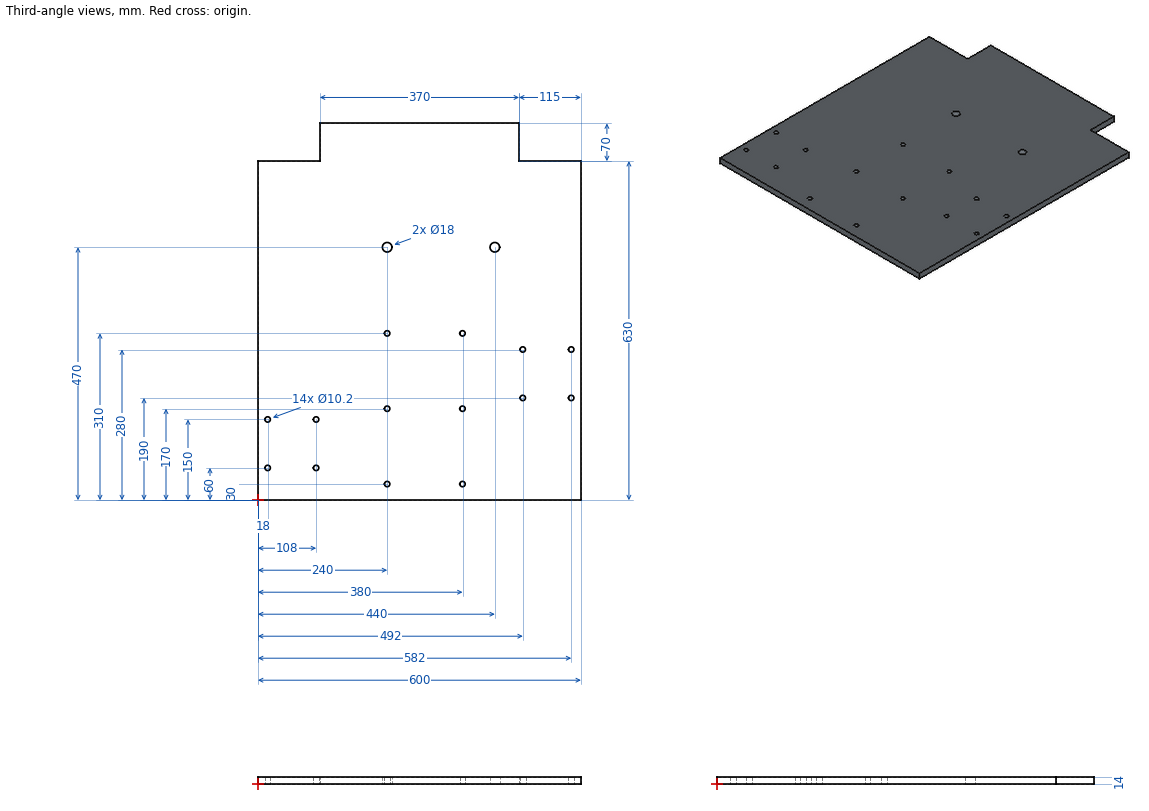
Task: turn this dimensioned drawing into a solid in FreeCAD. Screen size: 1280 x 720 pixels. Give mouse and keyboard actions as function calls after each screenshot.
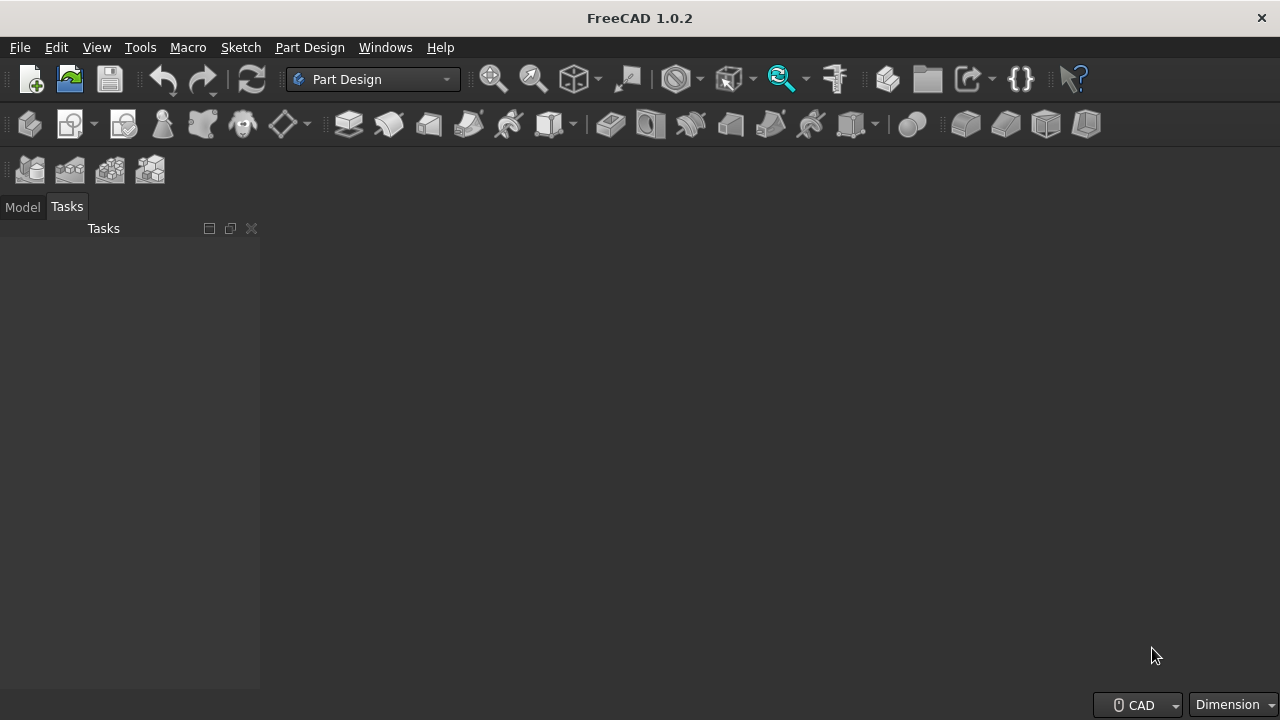
click(30, 80)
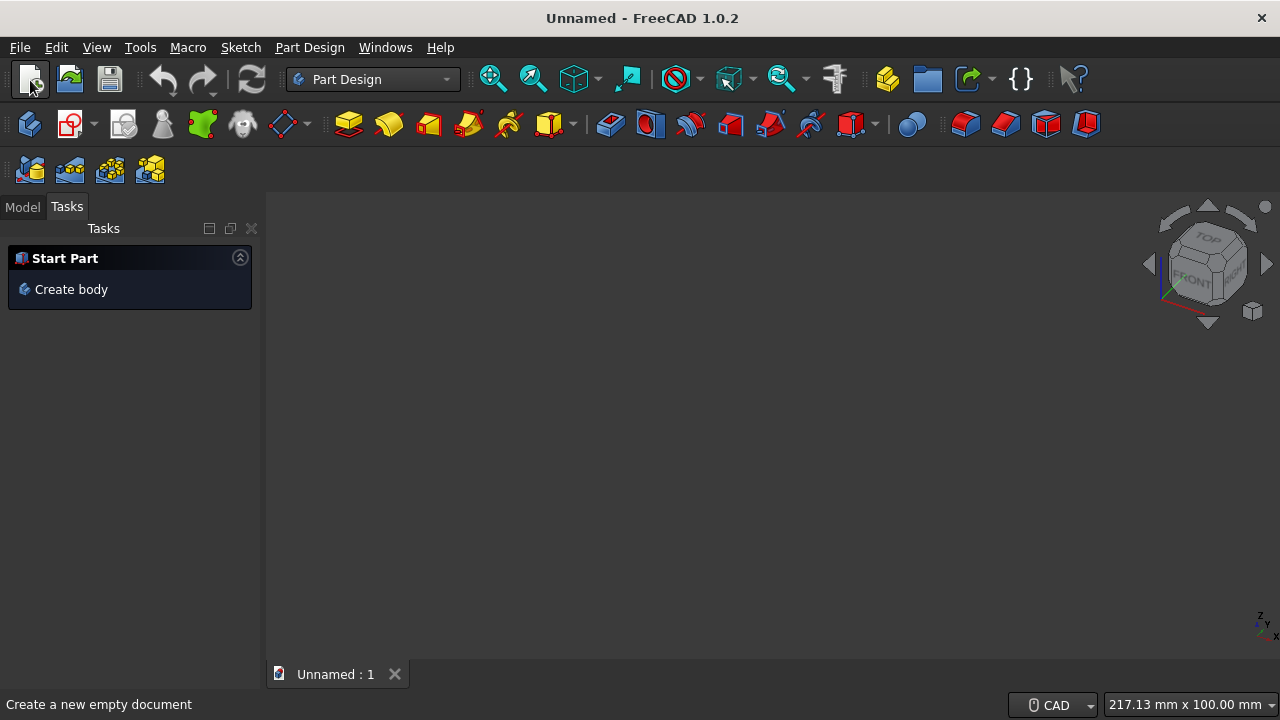
click(70, 124)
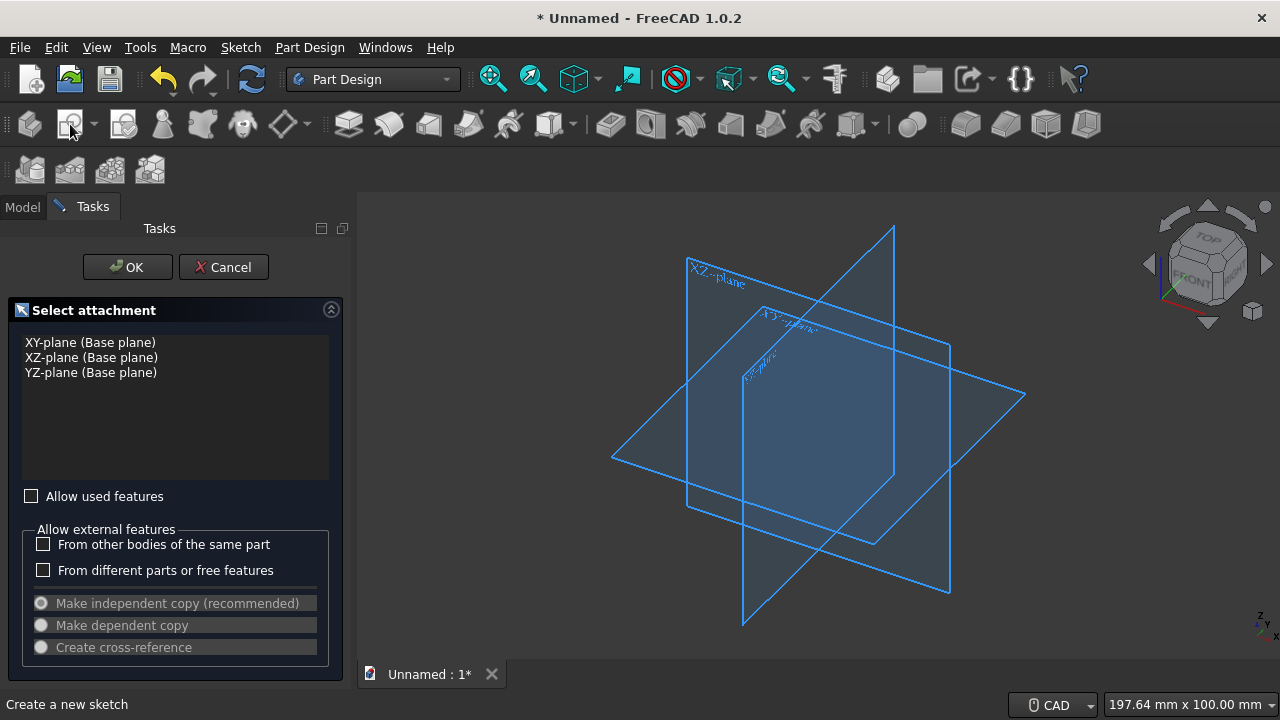
click(82, 342)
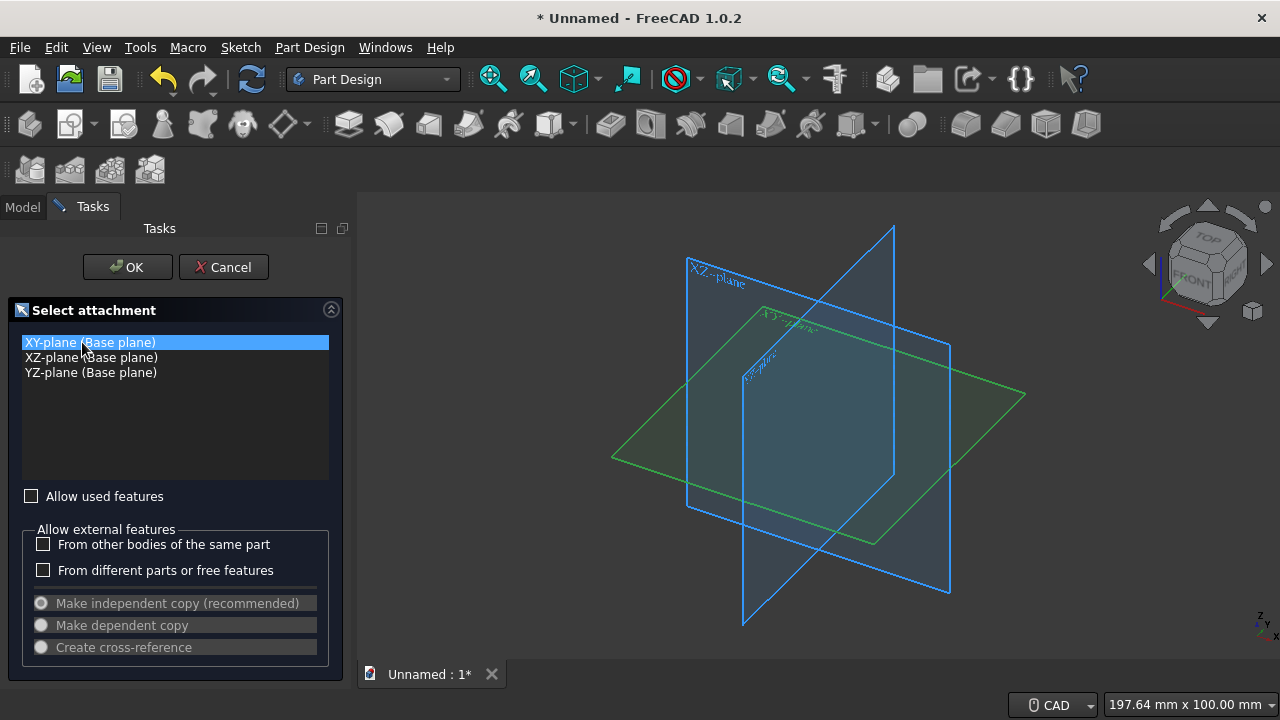
click(128, 267)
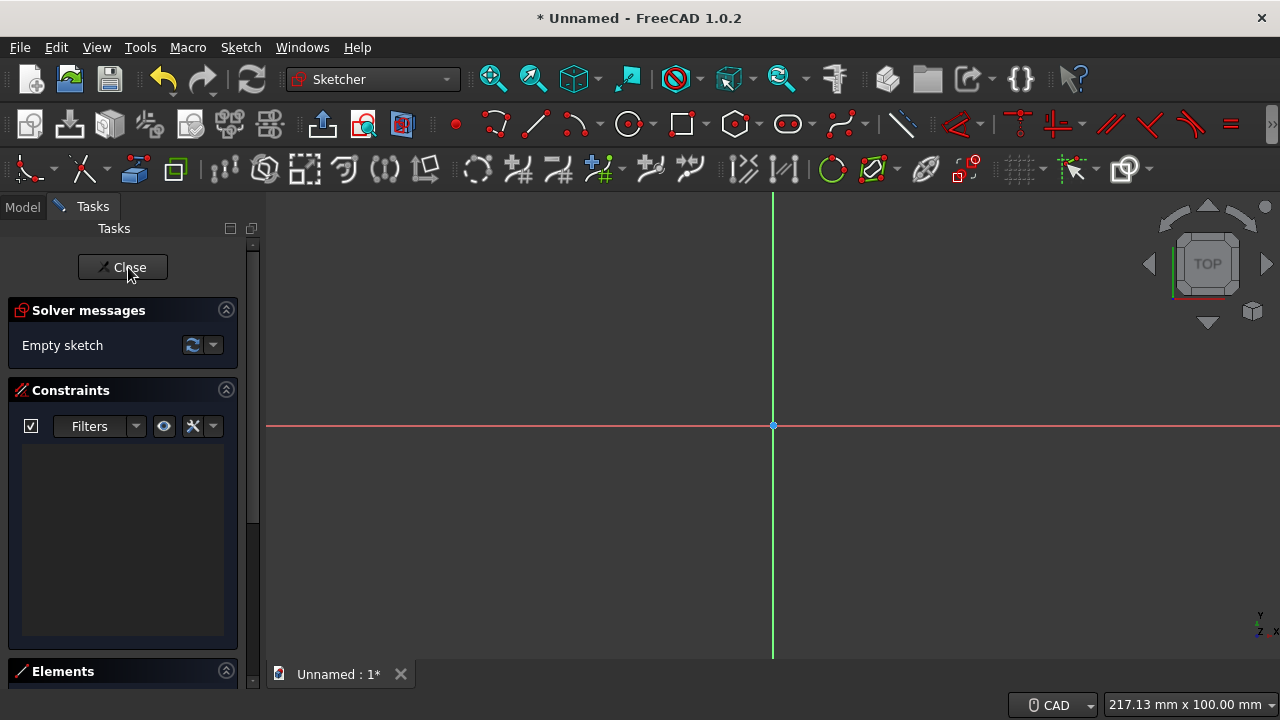
scroll(558, 589, down, 12)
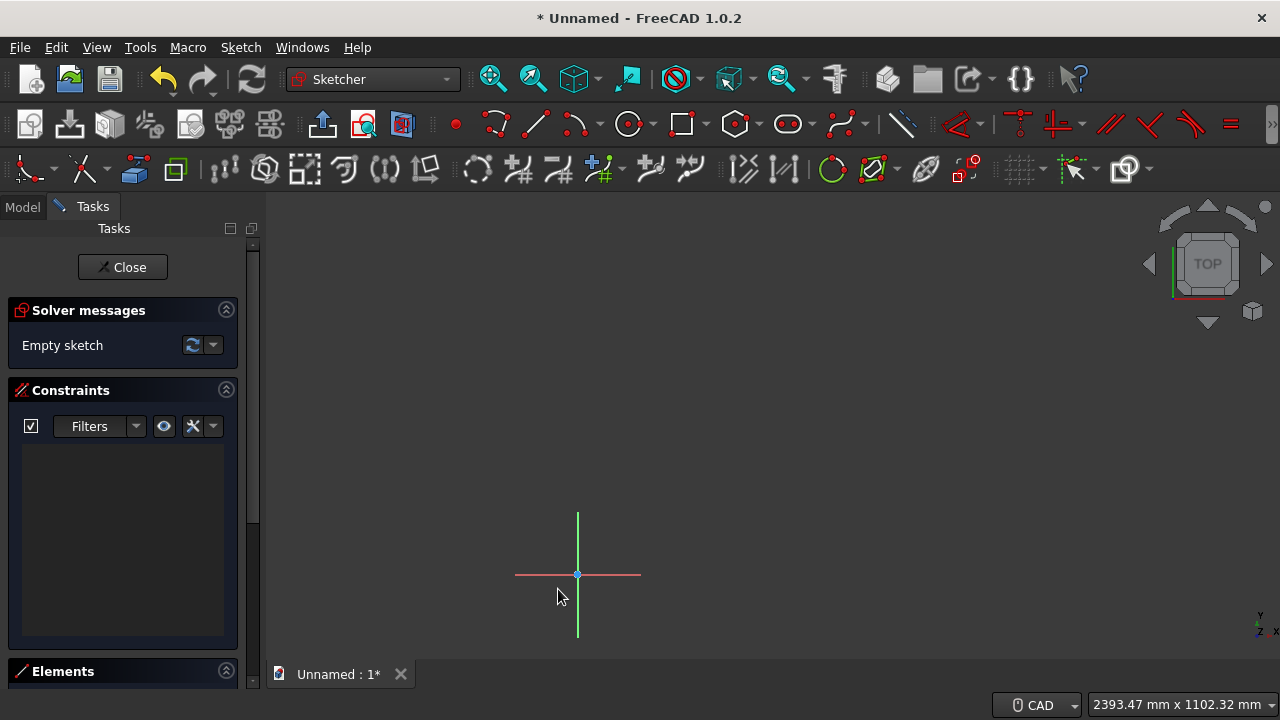
click(496, 124)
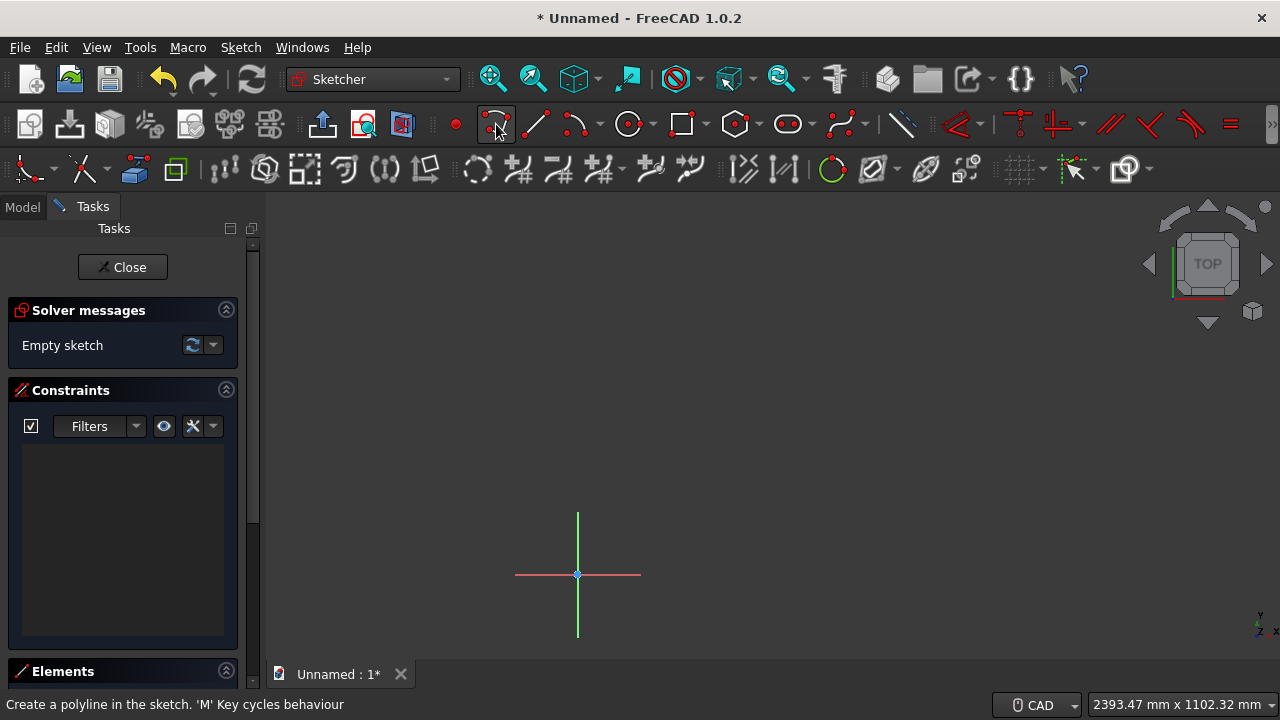
click(578, 575)
click(832, 566)
click(832, 308)
click(783, 308)
click(783, 278)
click(626, 278)
click(626, 308)
click(587, 308)
click(578, 575)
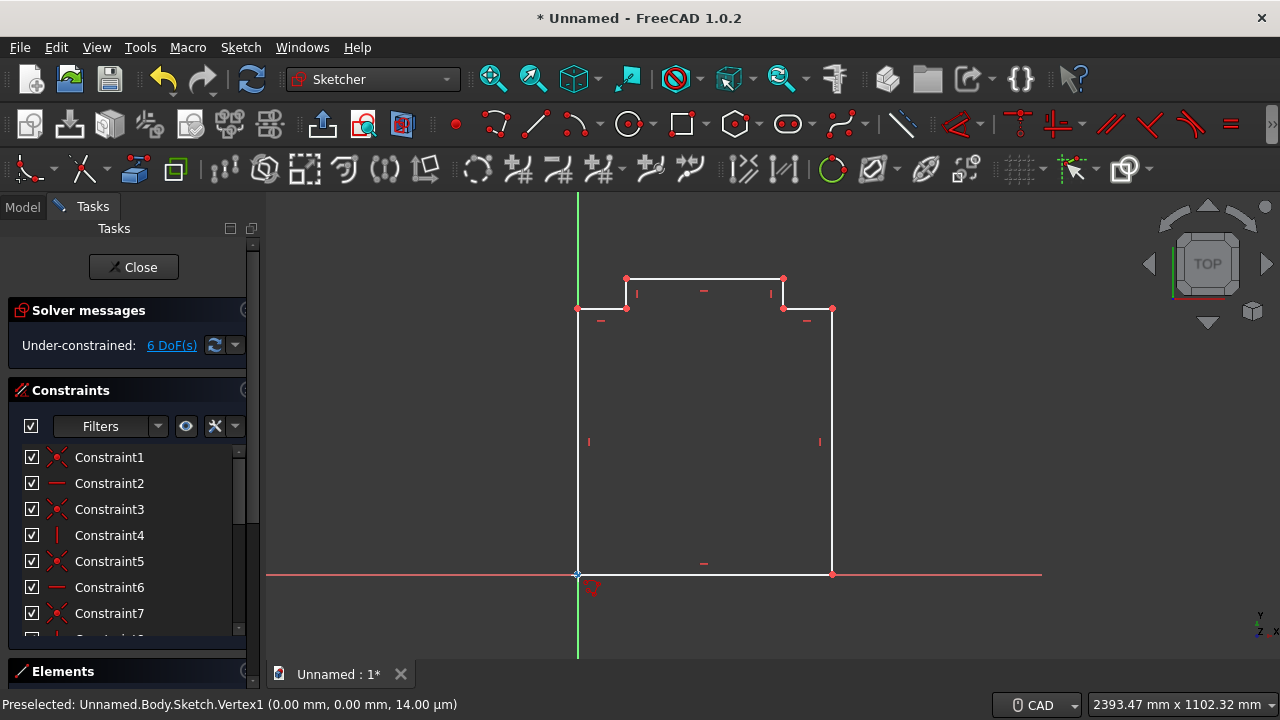
key(g)
key(c)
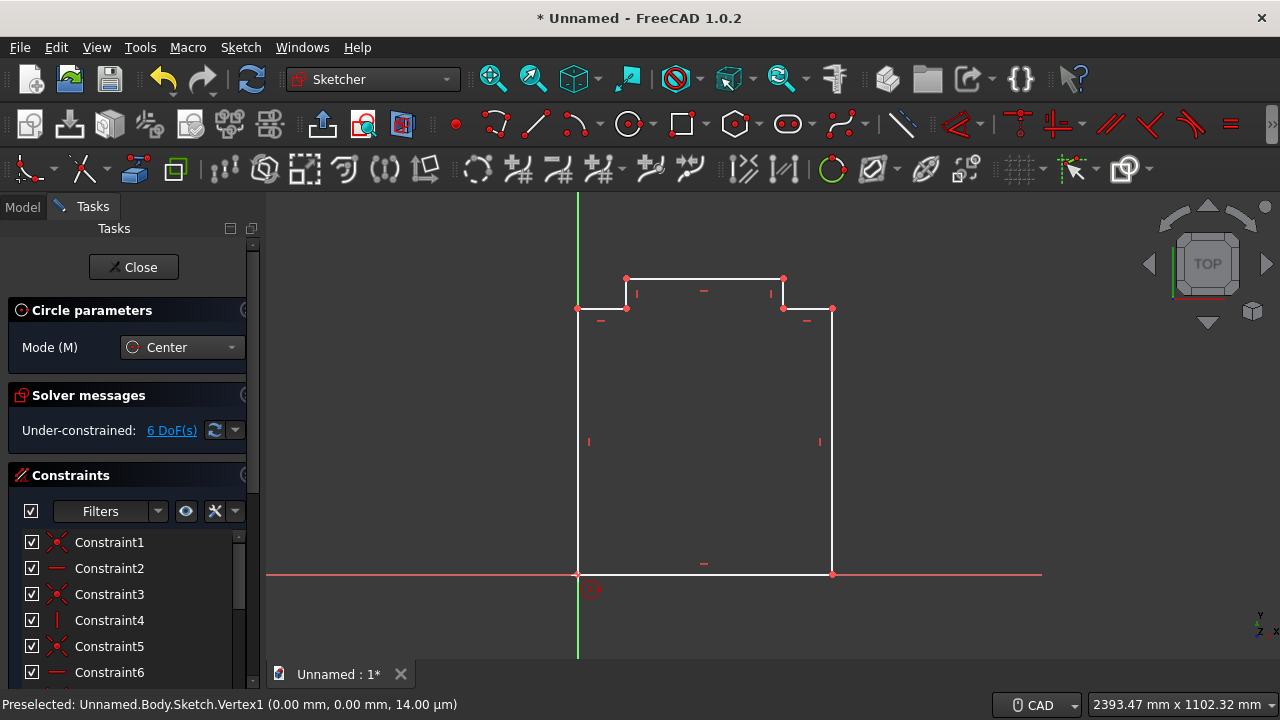
scroll(679, 376, up, 9)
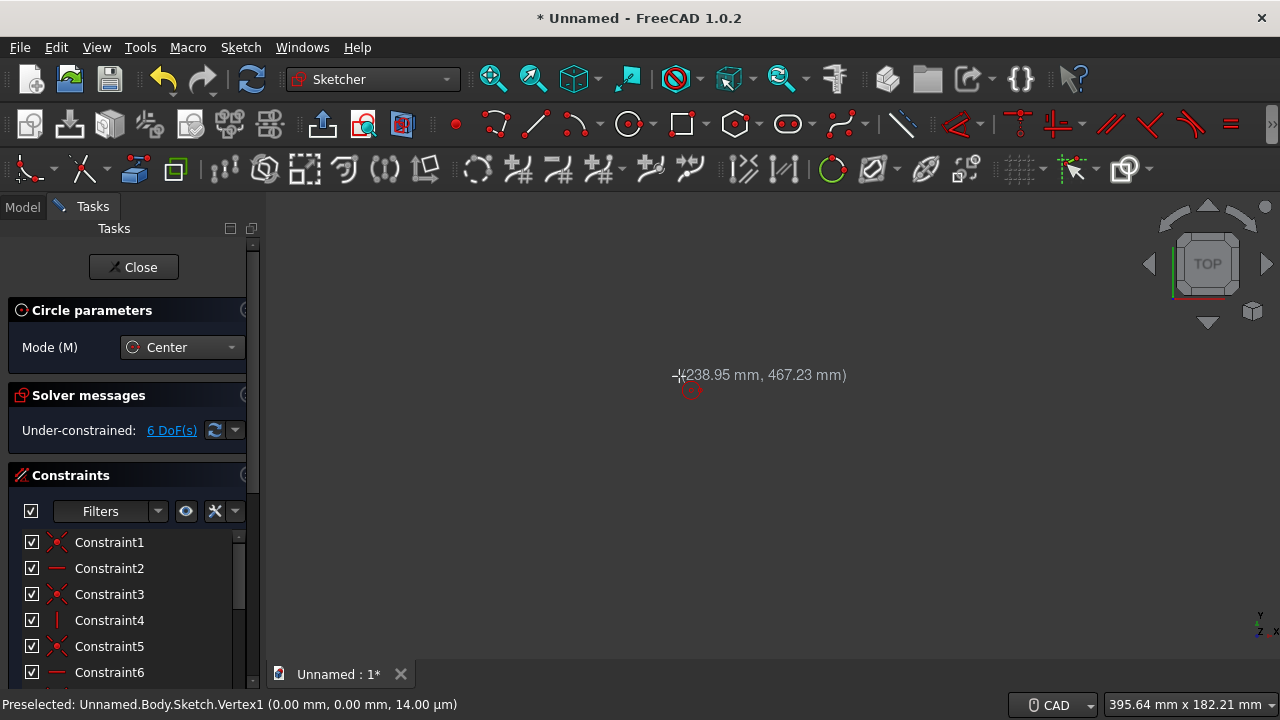
scroll(679, 375, down, 9)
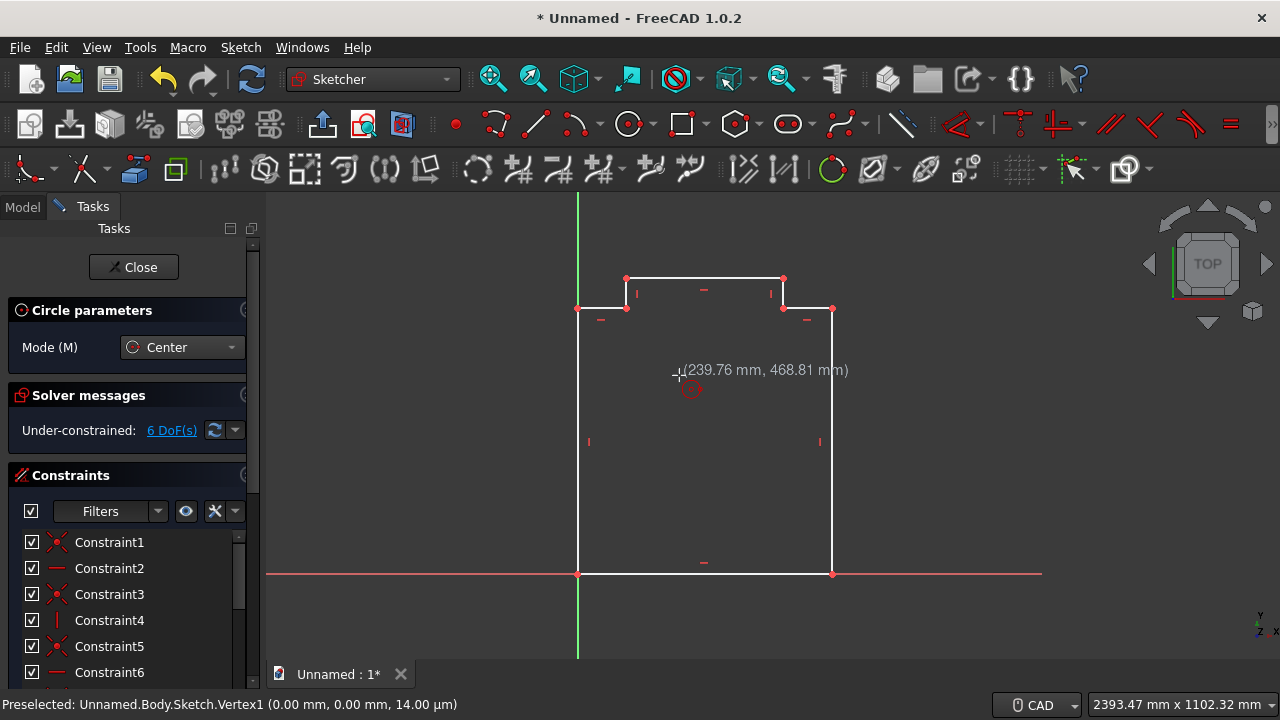
click(679, 375)